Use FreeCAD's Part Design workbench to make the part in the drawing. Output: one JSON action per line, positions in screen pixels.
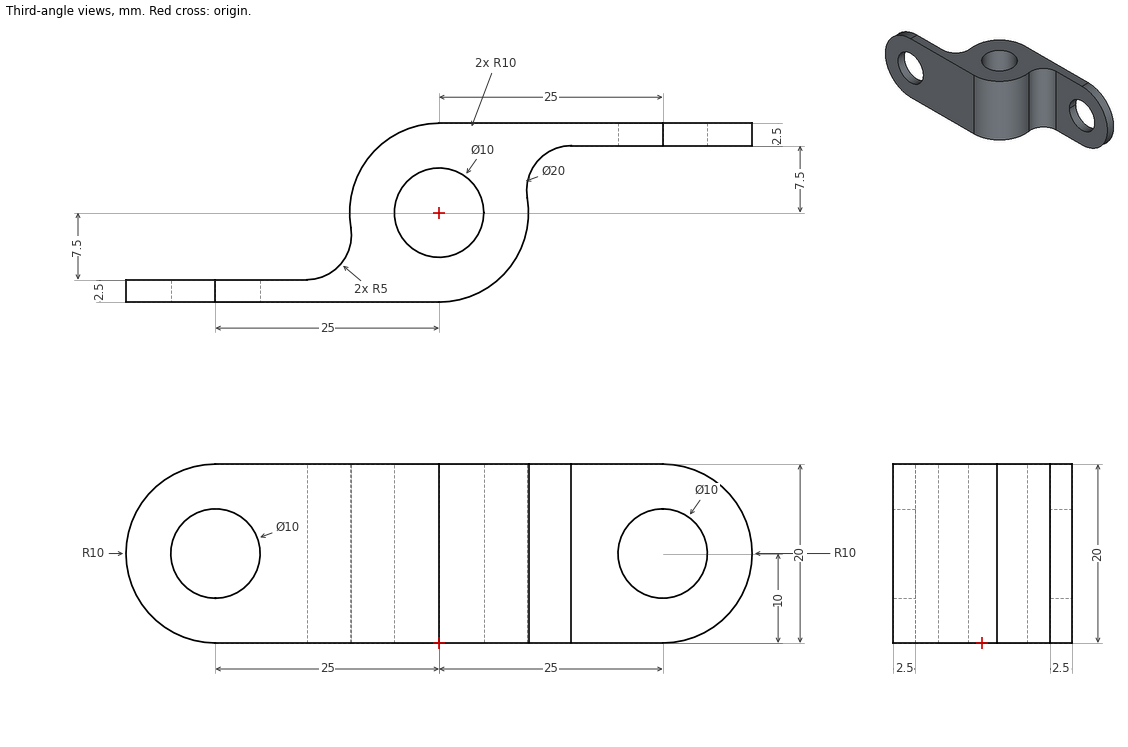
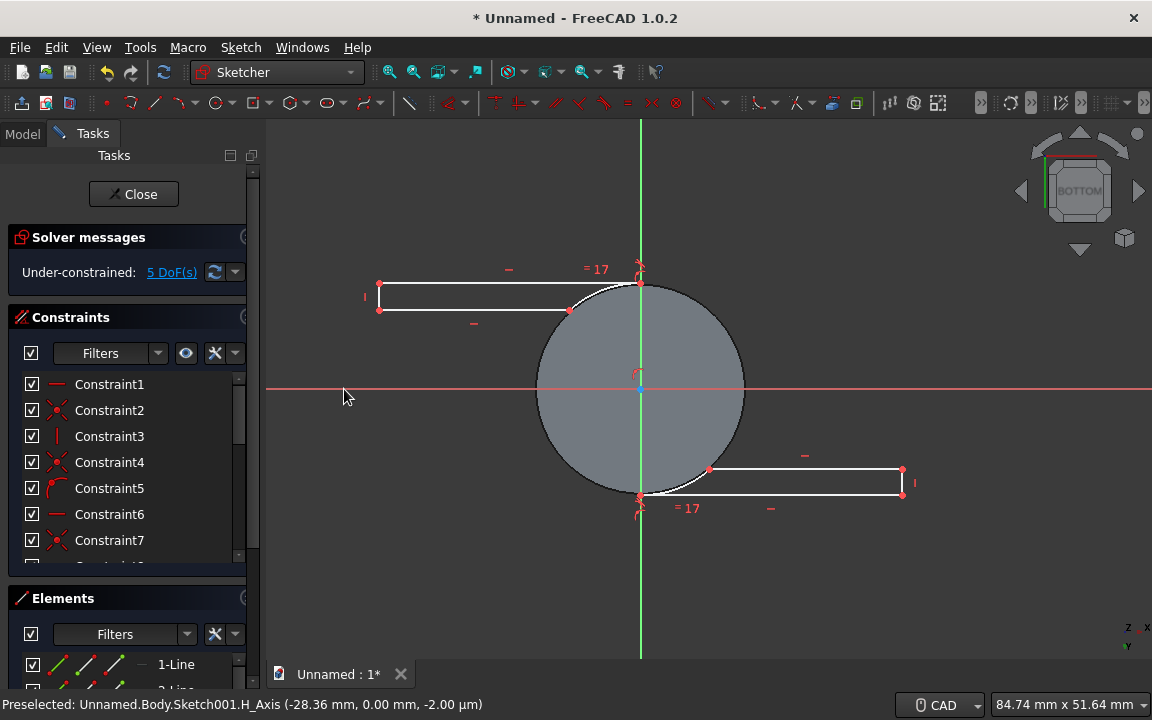
{"action": "left_click", "coordinate": [448, 104]}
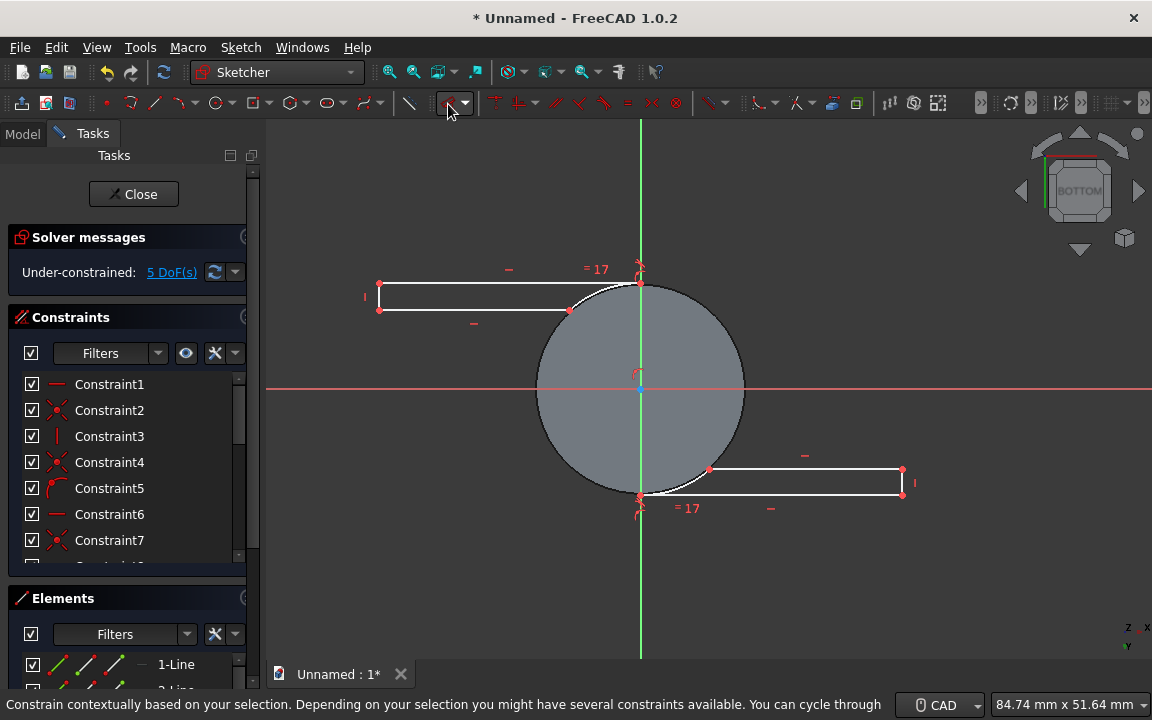
{"action": "left_click", "coordinate": [691, 482]}
{"action": "left_click", "coordinate": [706, 510]}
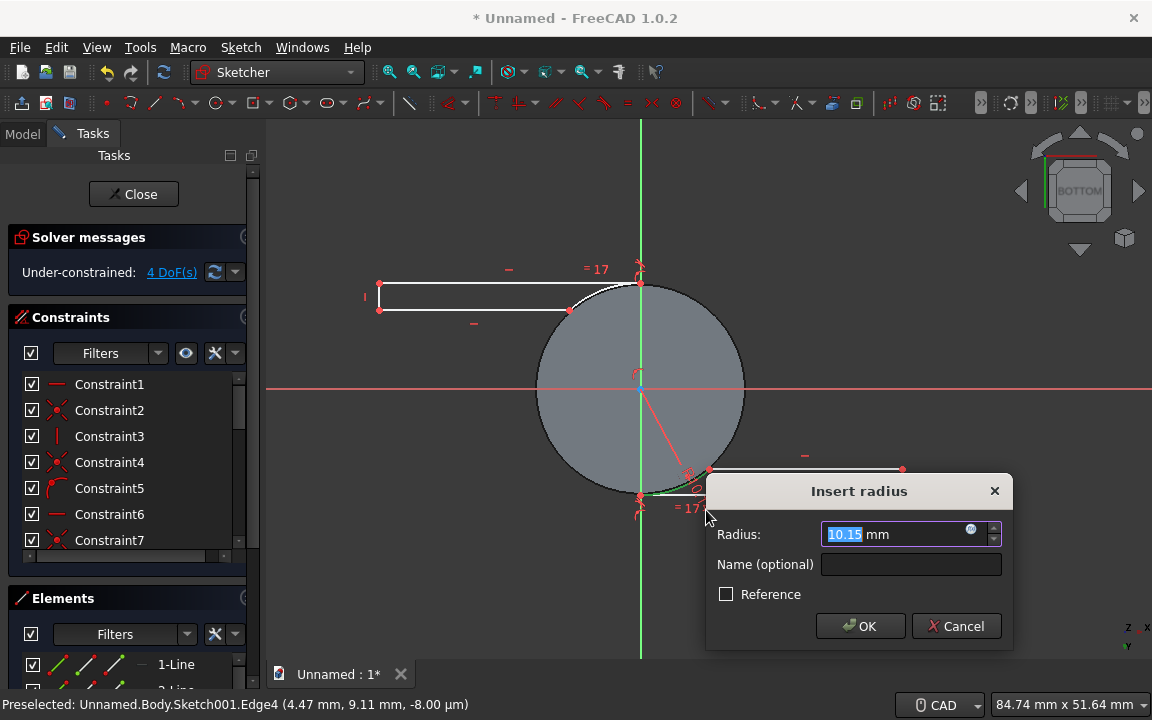
{"action": "type", "text": "10"}
{"action": "key", "text": "Return"}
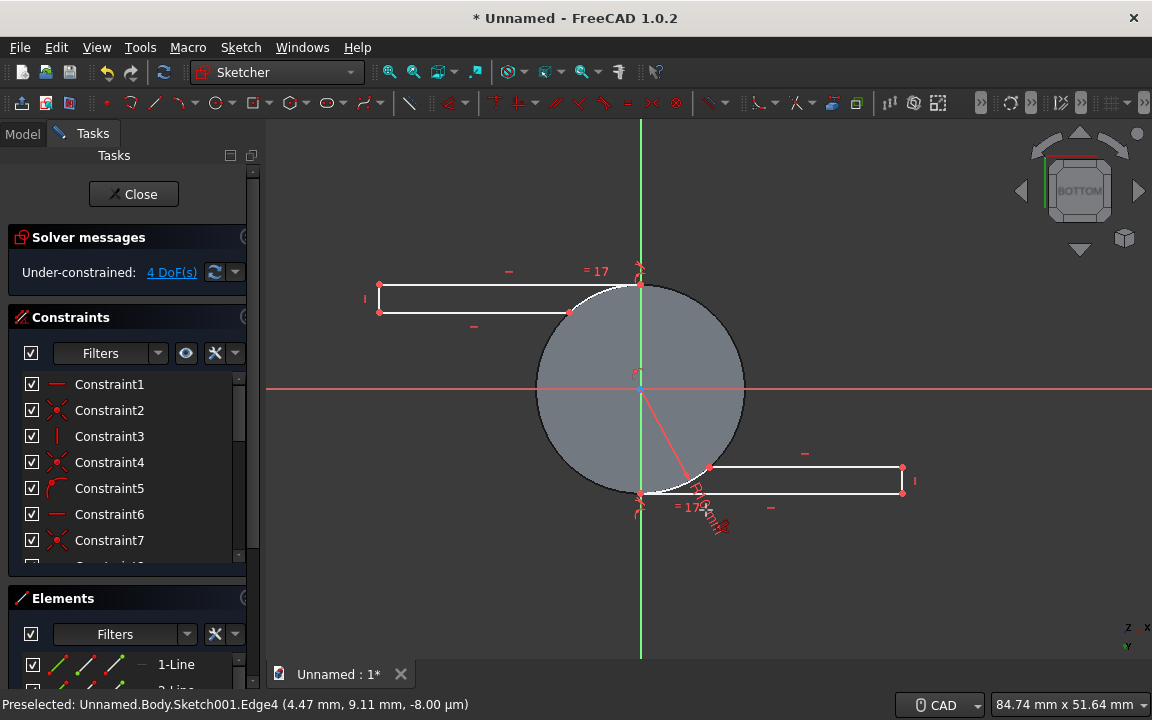
{"action": "left_click", "coordinate": [824, 494]}
{"action": "left_click", "coordinate": [831, 528]}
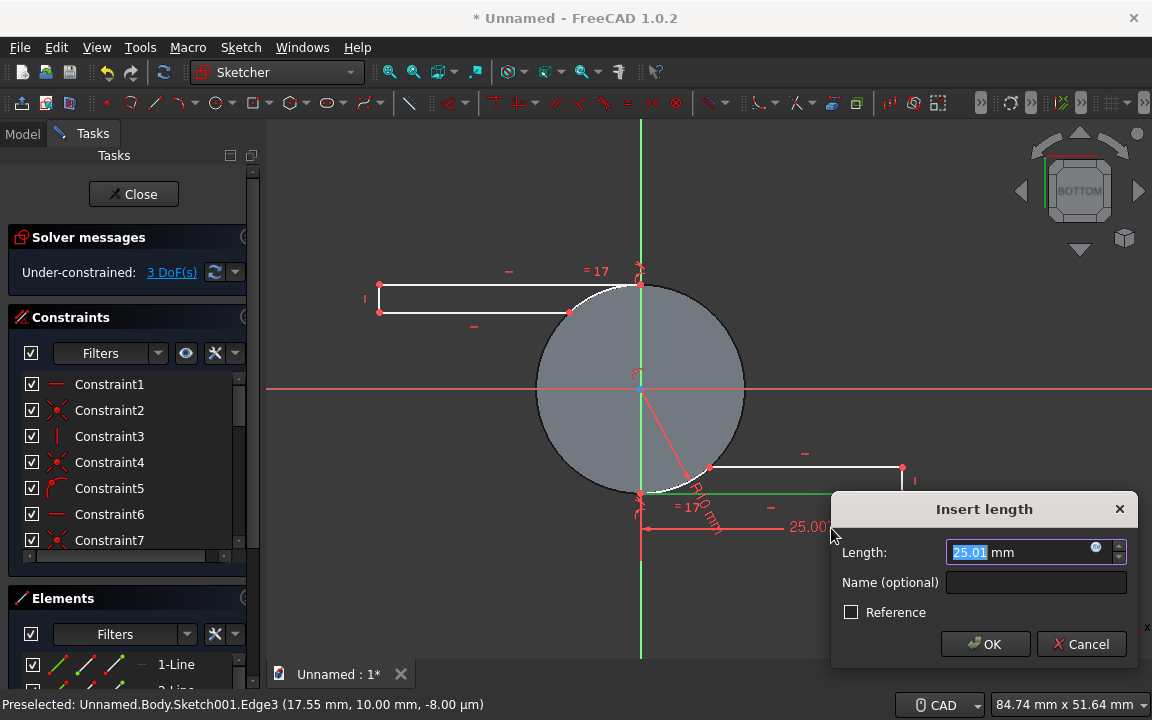
{"action": "type", "text": "25"}
{"action": "key", "text": "Return"}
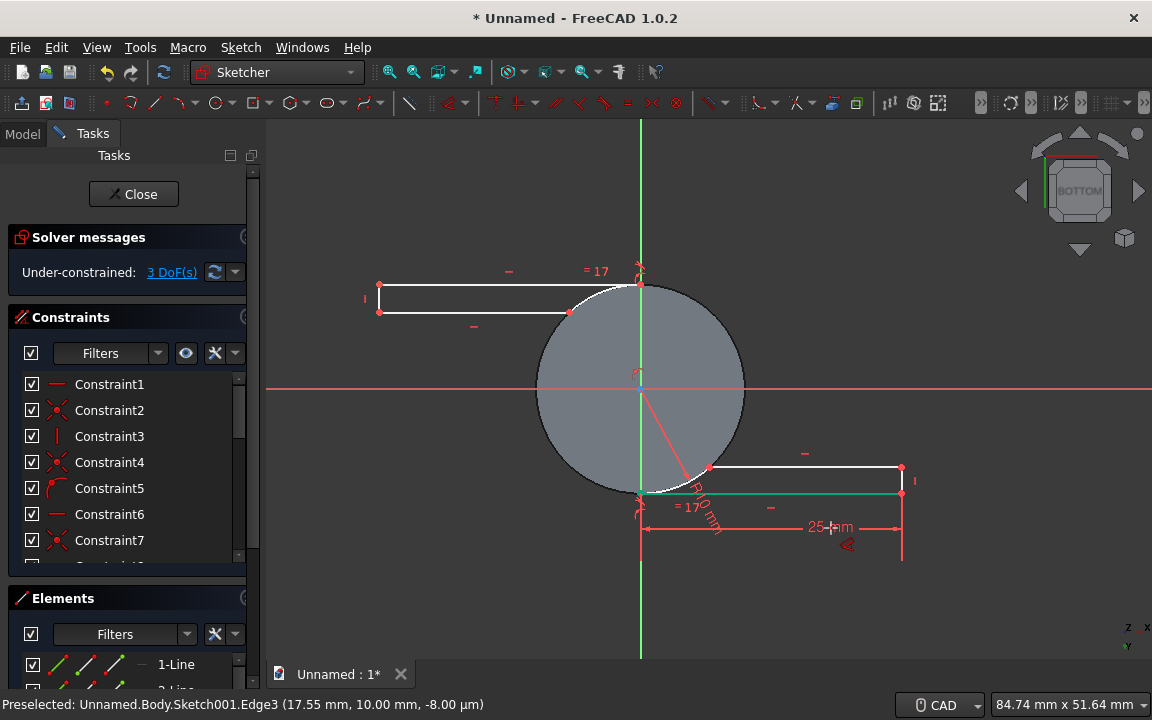
{"action": "left_click", "coordinate": [457, 285]}
{"action": "left_click", "coordinate": [510, 251]}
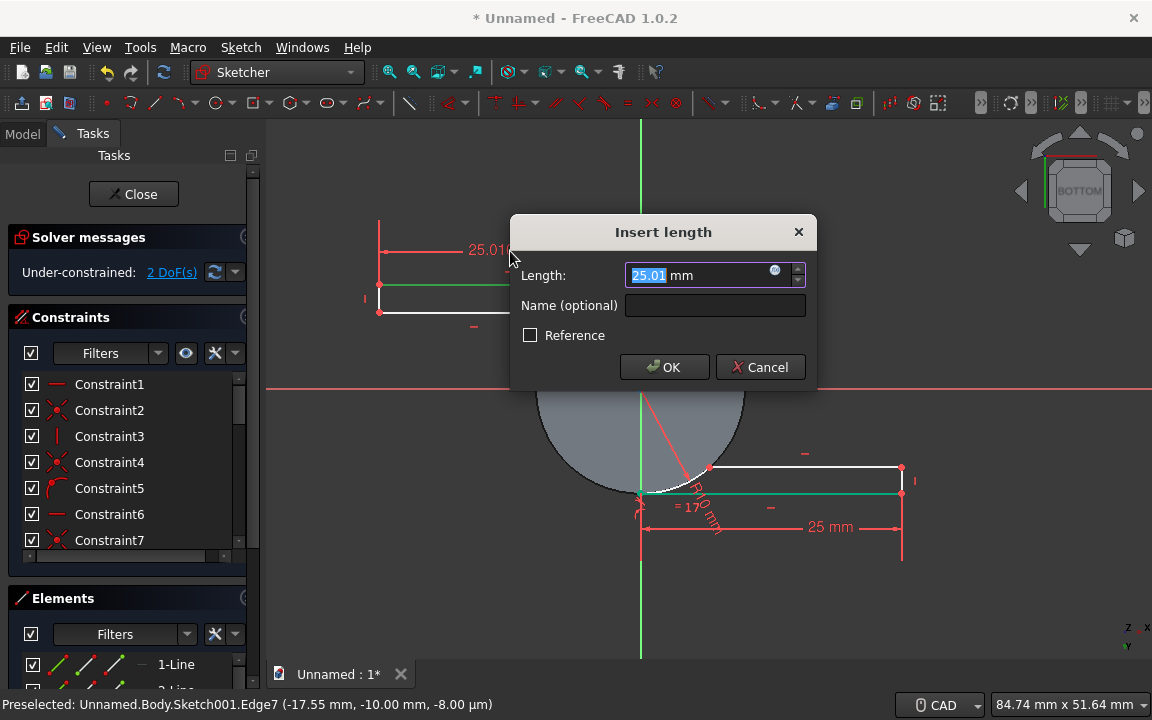
{"action": "type", "text": "25"}
{"action": "key", "text": "Return"}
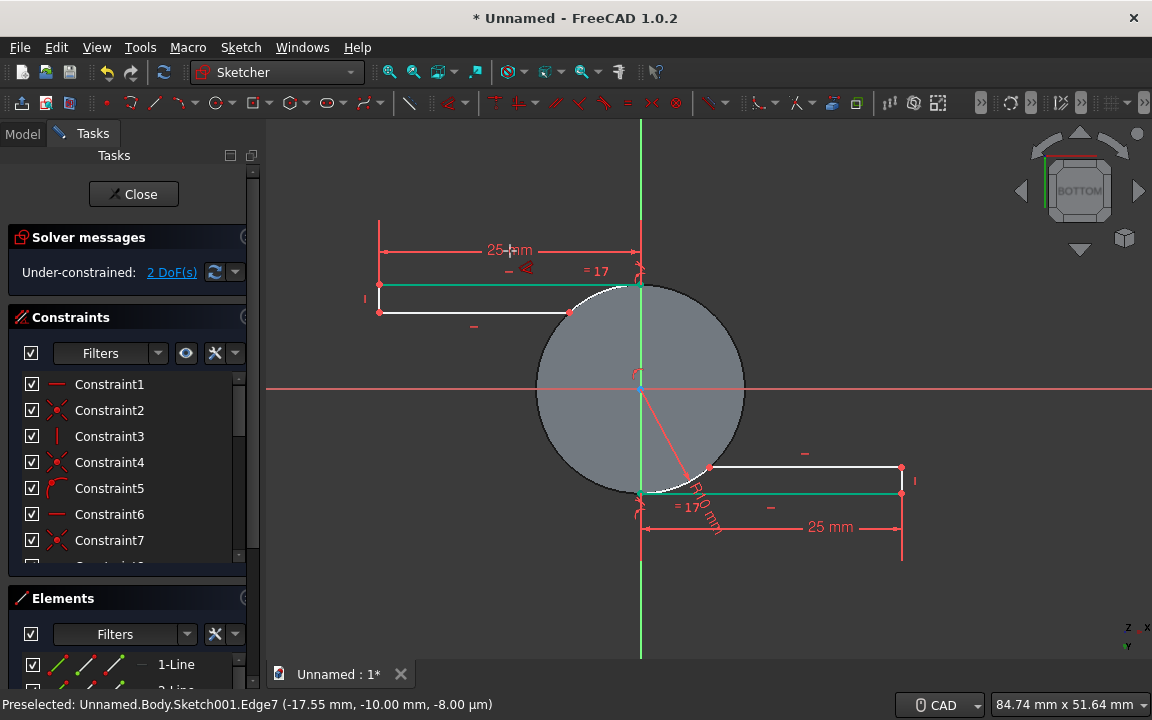
{"action": "scroll", "coordinate": [902, 478], "scroll_direction": "up", "scroll_amount": 3}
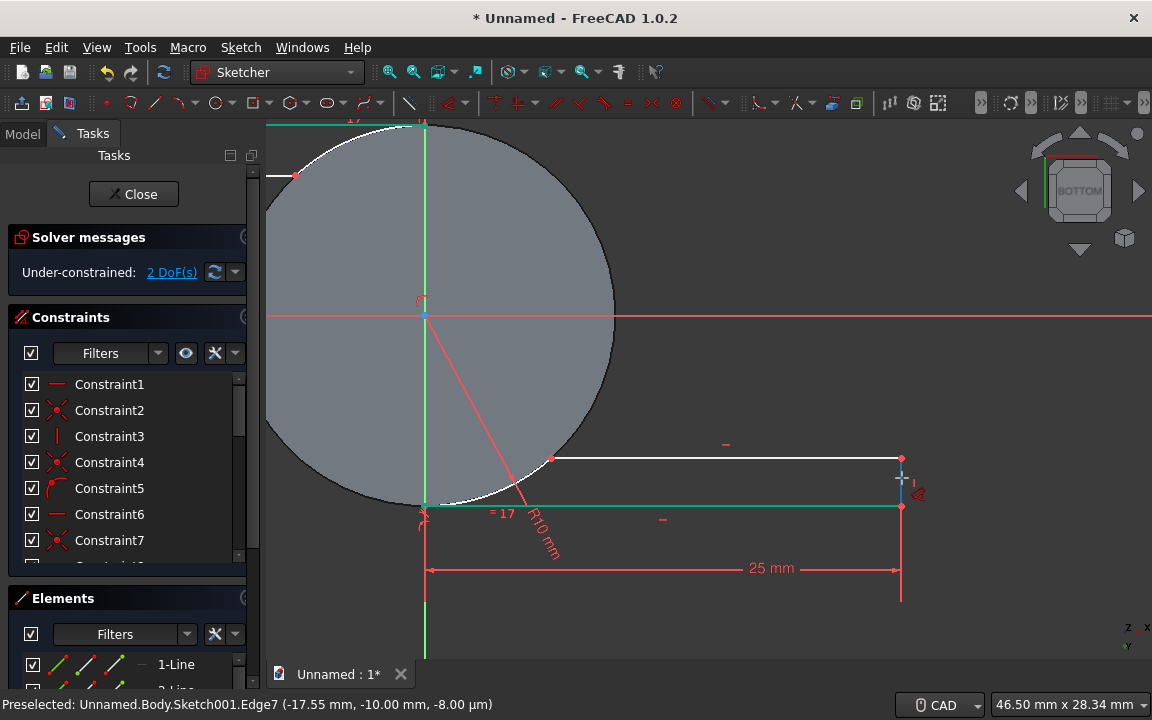
{"action": "left_click", "coordinate": [901, 477]}
{"action": "left_click", "coordinate": [935, 482]}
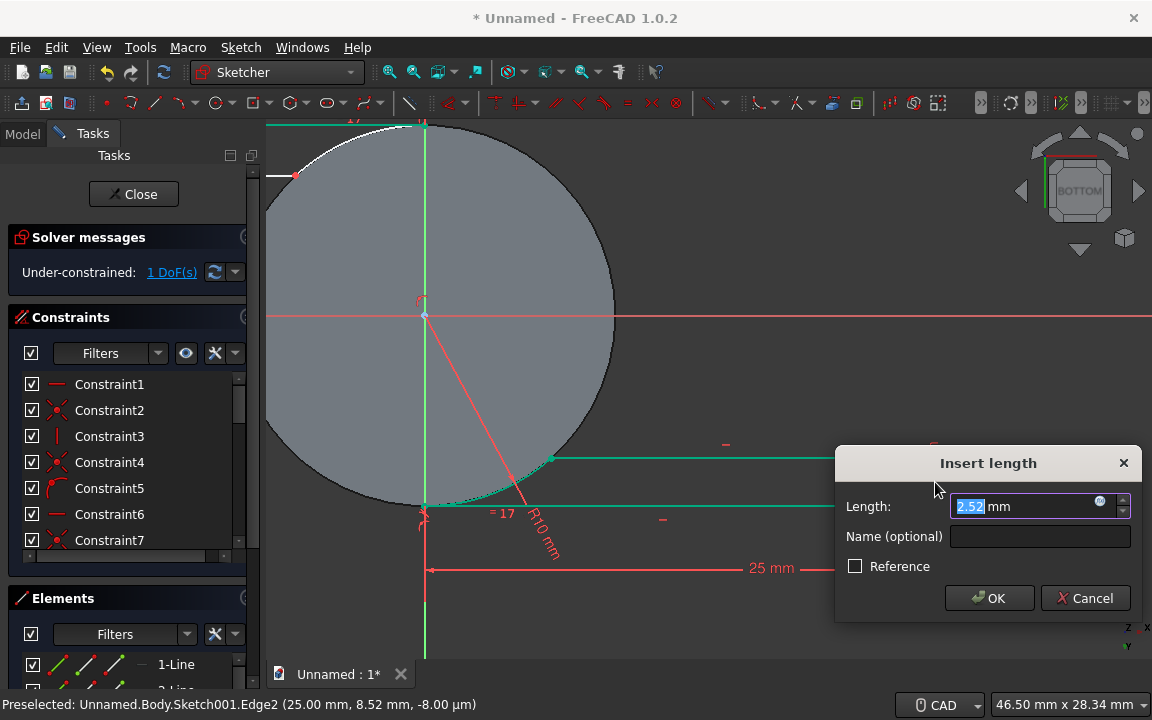
{"action": "type", "text": "2.5"}
{"action": "key", "text": "Return"}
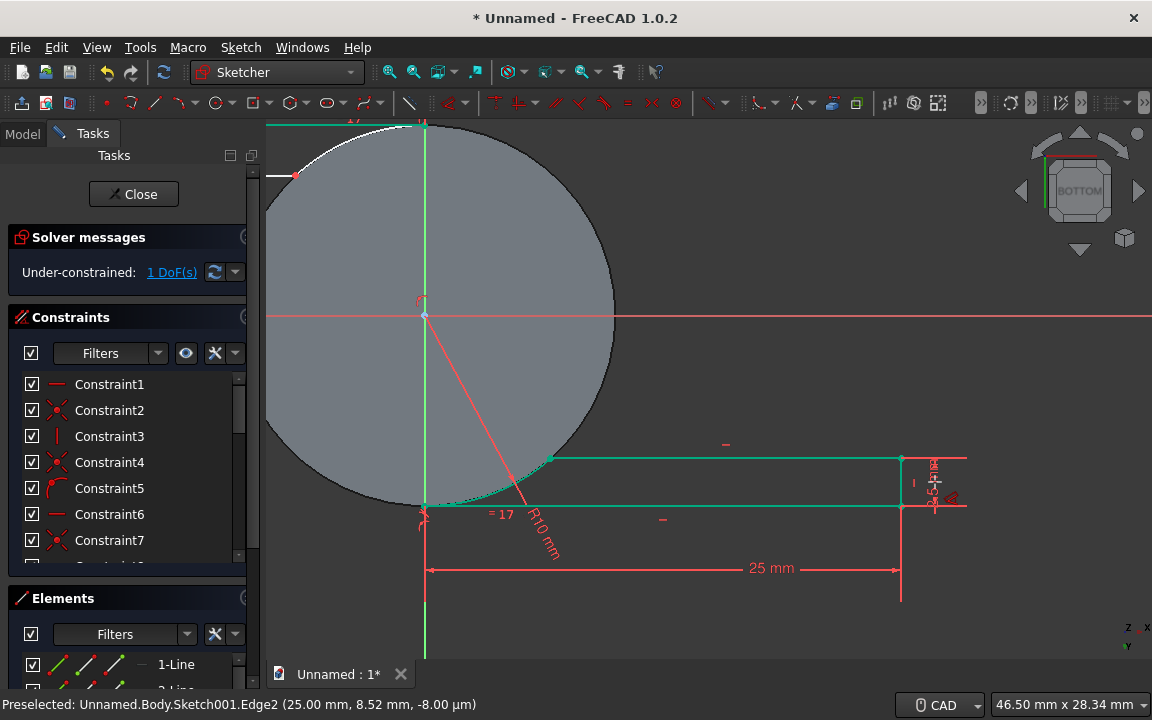
{"action": "scroll", "coordinate": [903, 478], "scroll_direction": "down", "scroll_amount": 3}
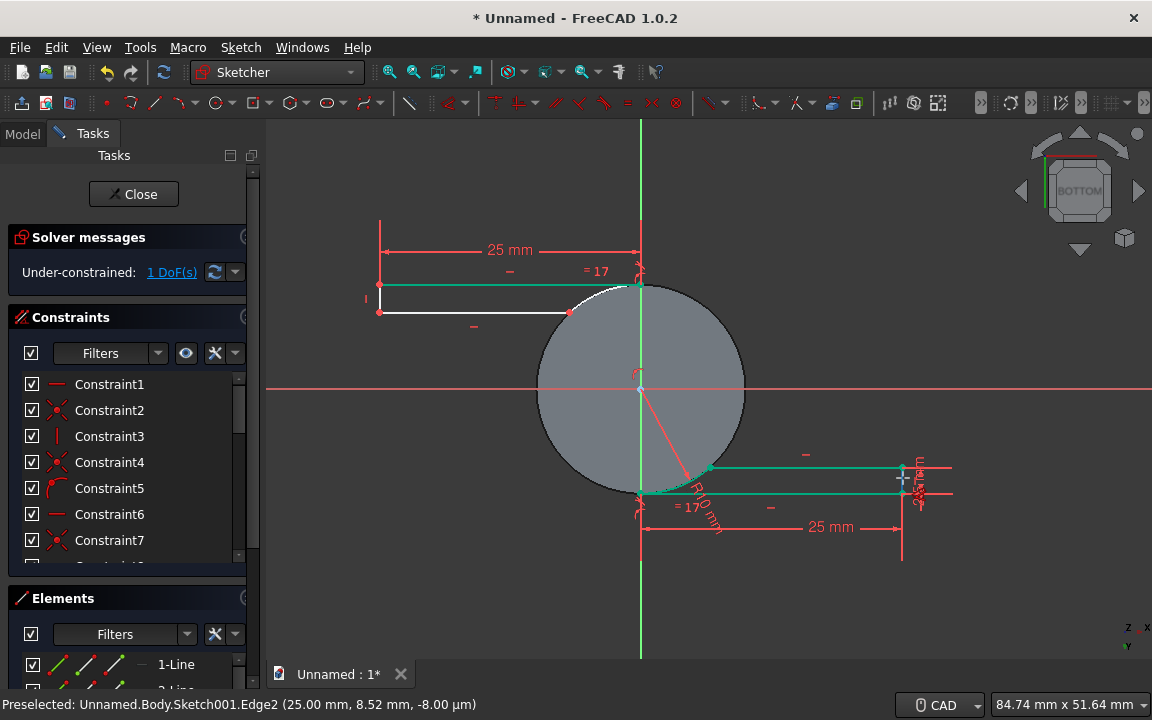
{"action": "scroll", "coordinate": [380, 304], "scroll_direction": "up", "scroll_amount": 3}